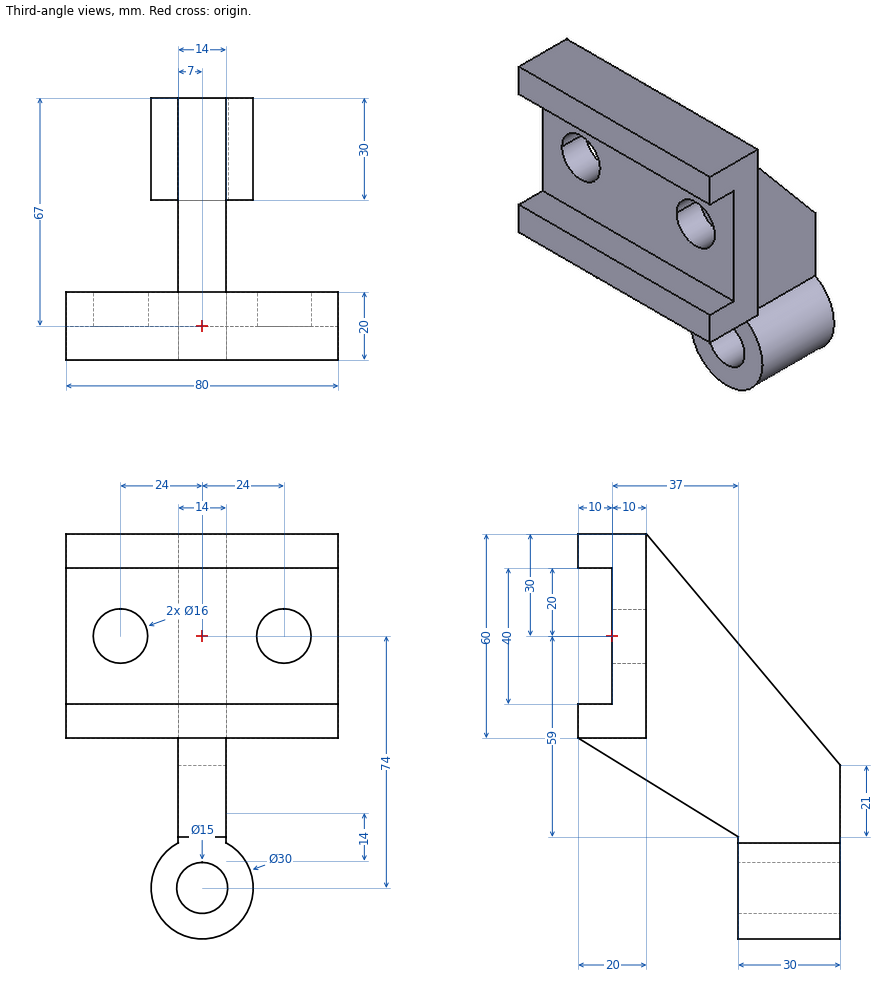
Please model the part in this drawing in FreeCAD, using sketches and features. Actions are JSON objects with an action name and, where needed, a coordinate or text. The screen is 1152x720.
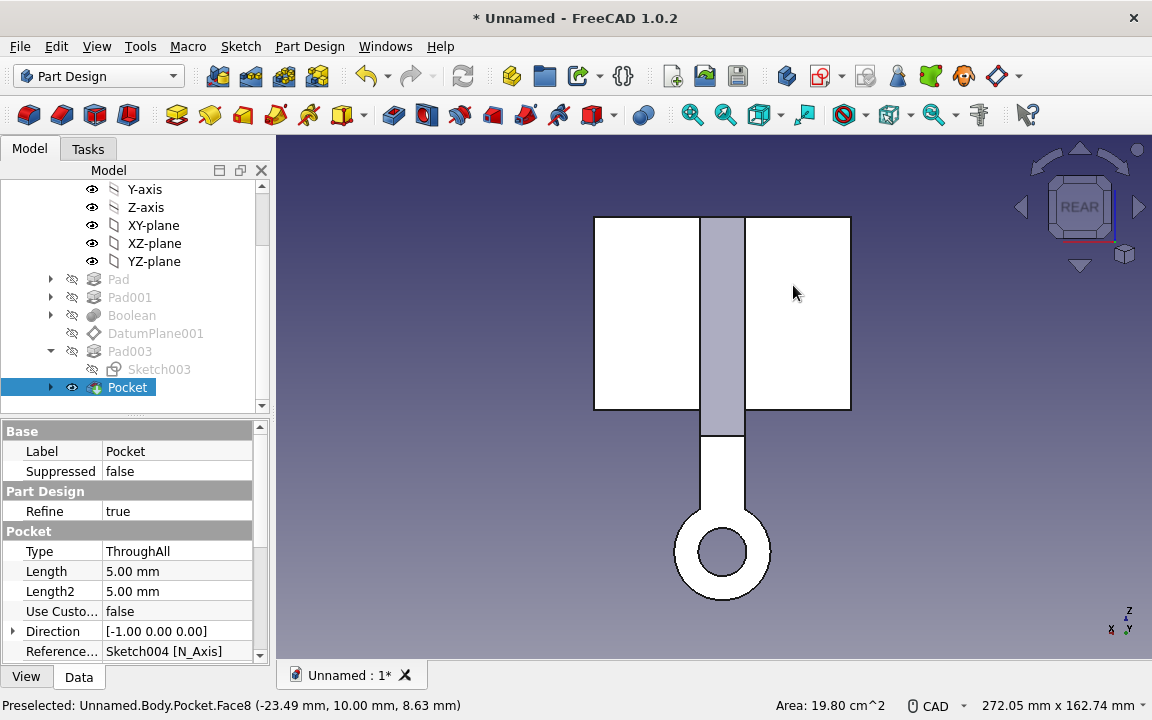
{"action": "left_click", "coordinate": [820, 76]}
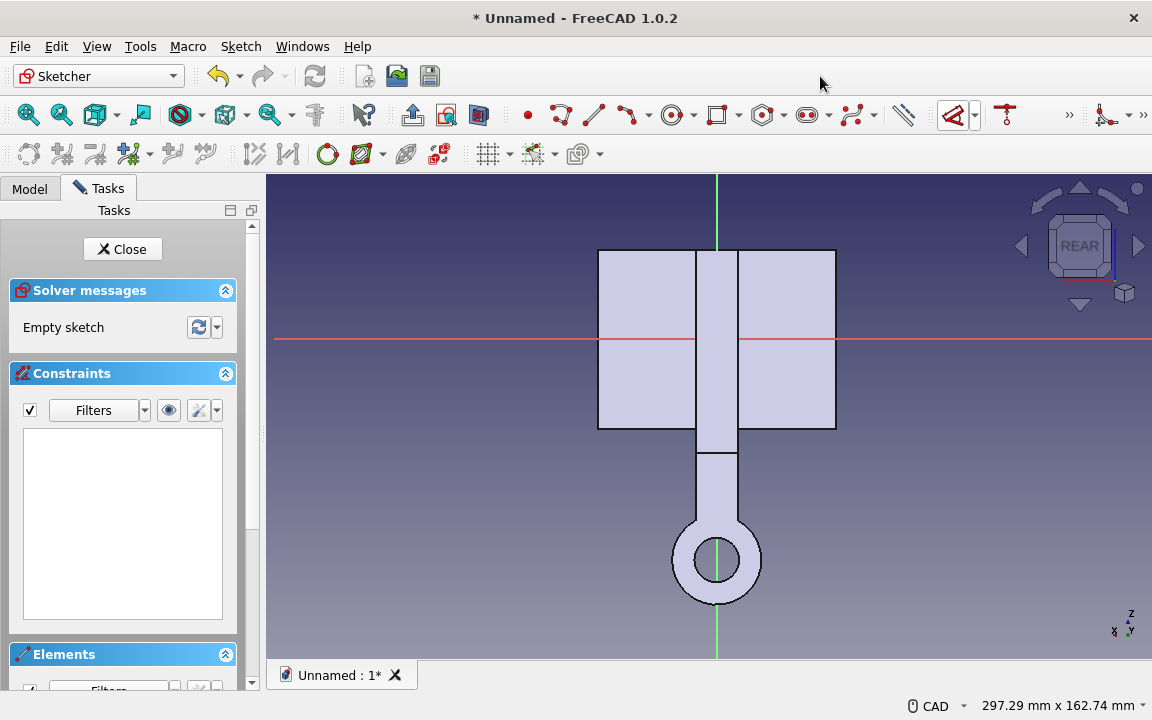
{"action": "scroll", "coordinate": [761, 295], "scroll_direction": "up", "scroll_amount": 5}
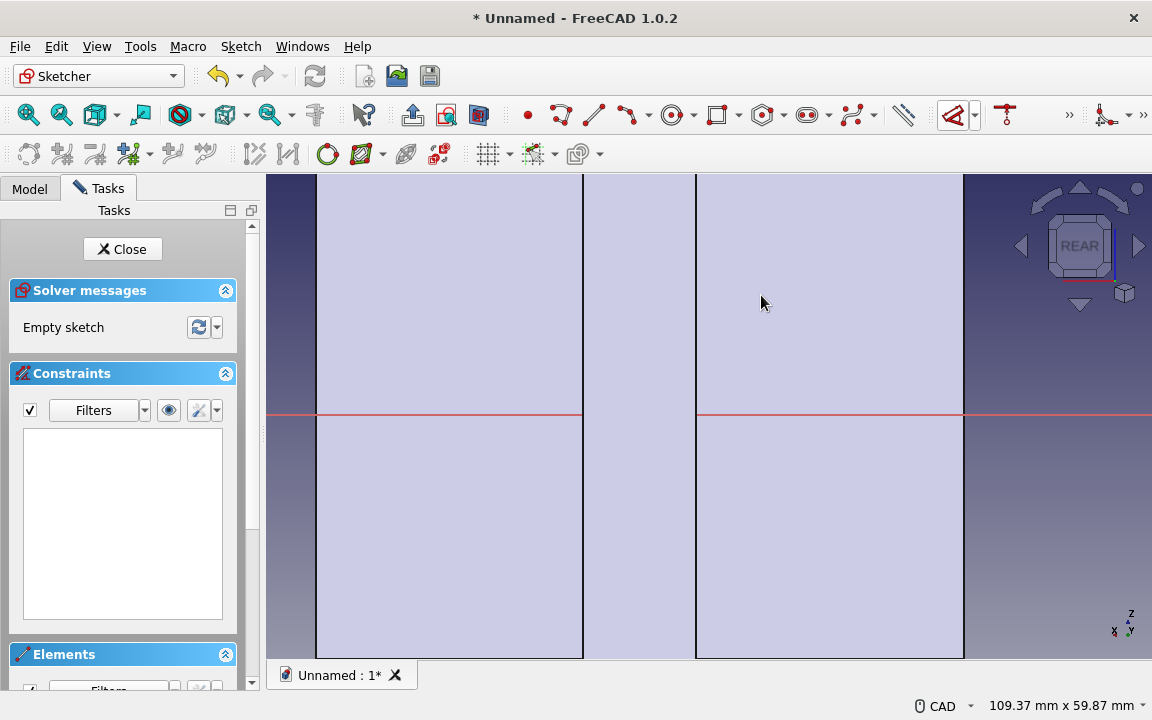
{"action": "left_click", "coordinate": [672, 116]}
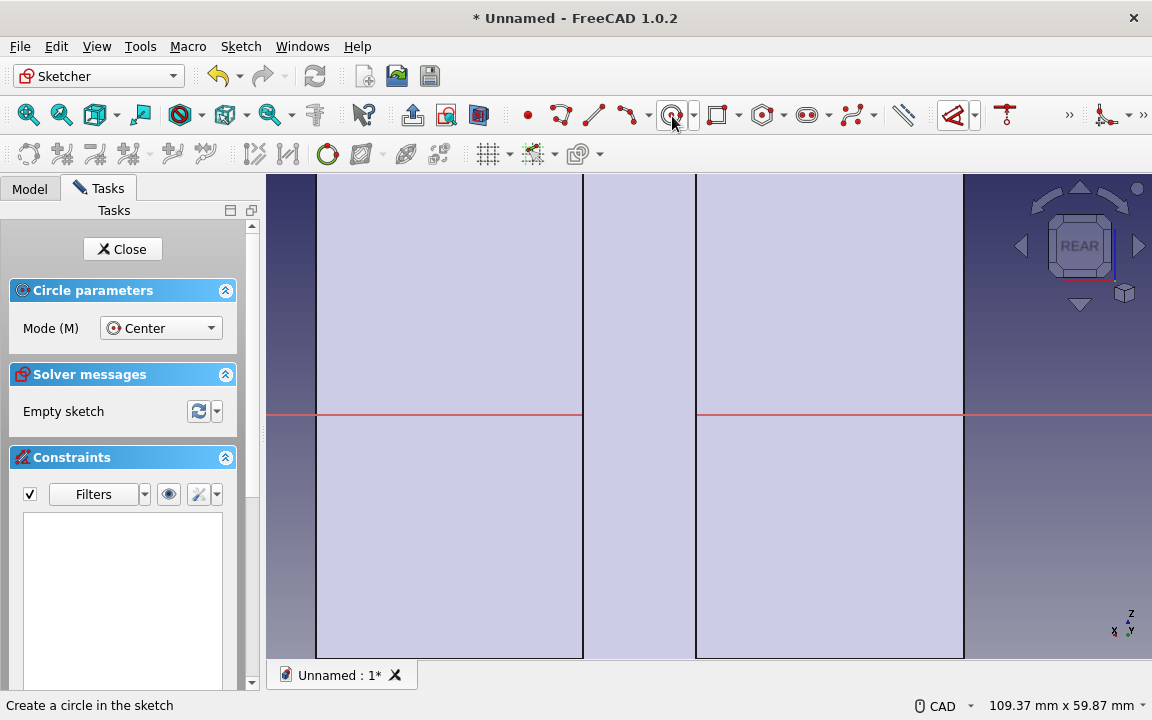
{"action": "left_click", "coordinate": [834, 415]}
{"action": "mouse_move", "coordinate": [880, 370]}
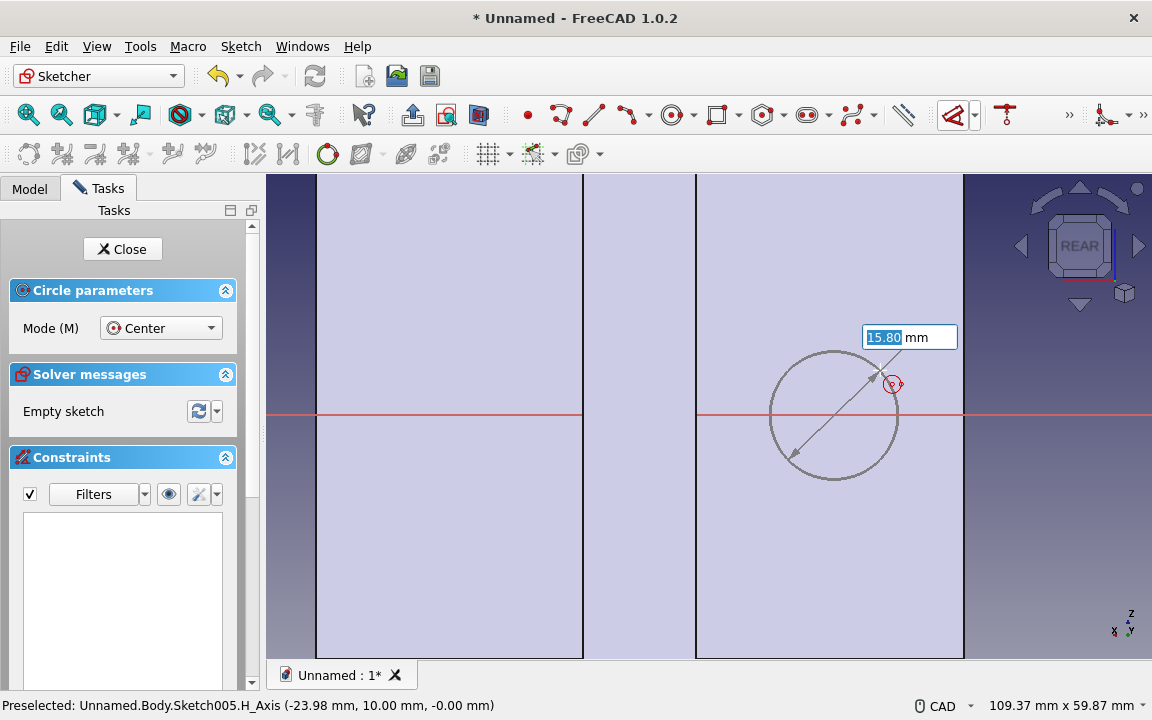
{"action": "type", "text": "16"}
{"action": "key", "text": "Return"}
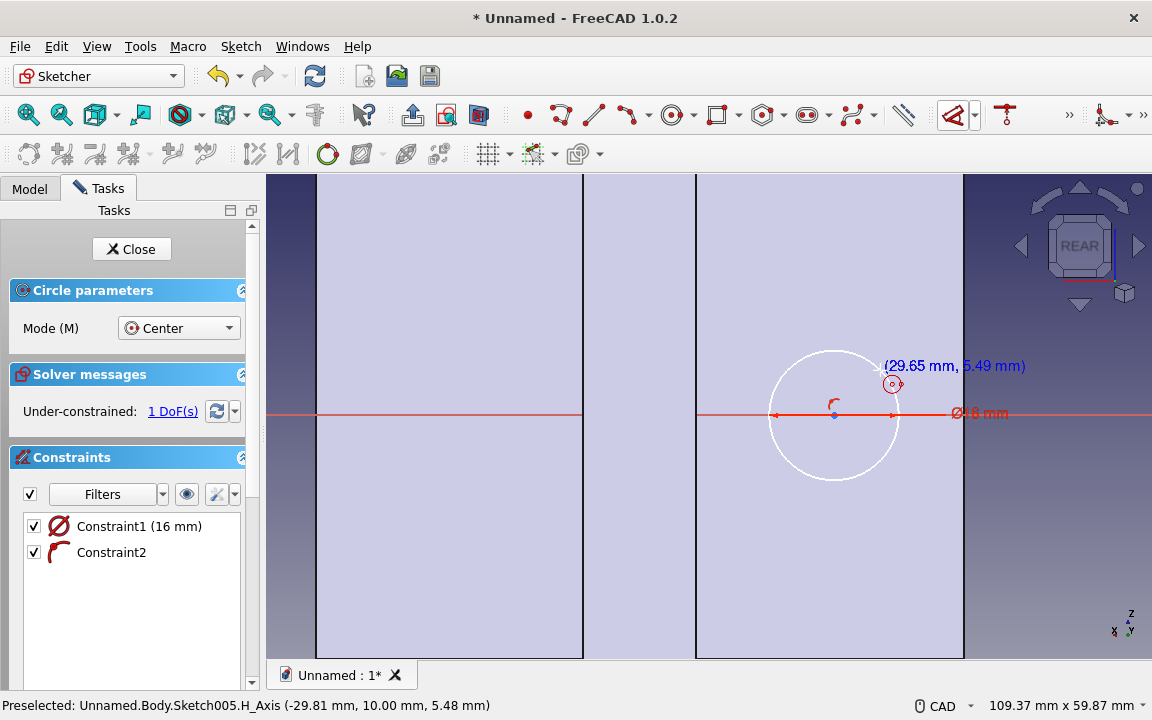
{"action": "left_click", "coordinate": [445, 415]}
{"action": "mouse_move", "coordinate": [491, 370]}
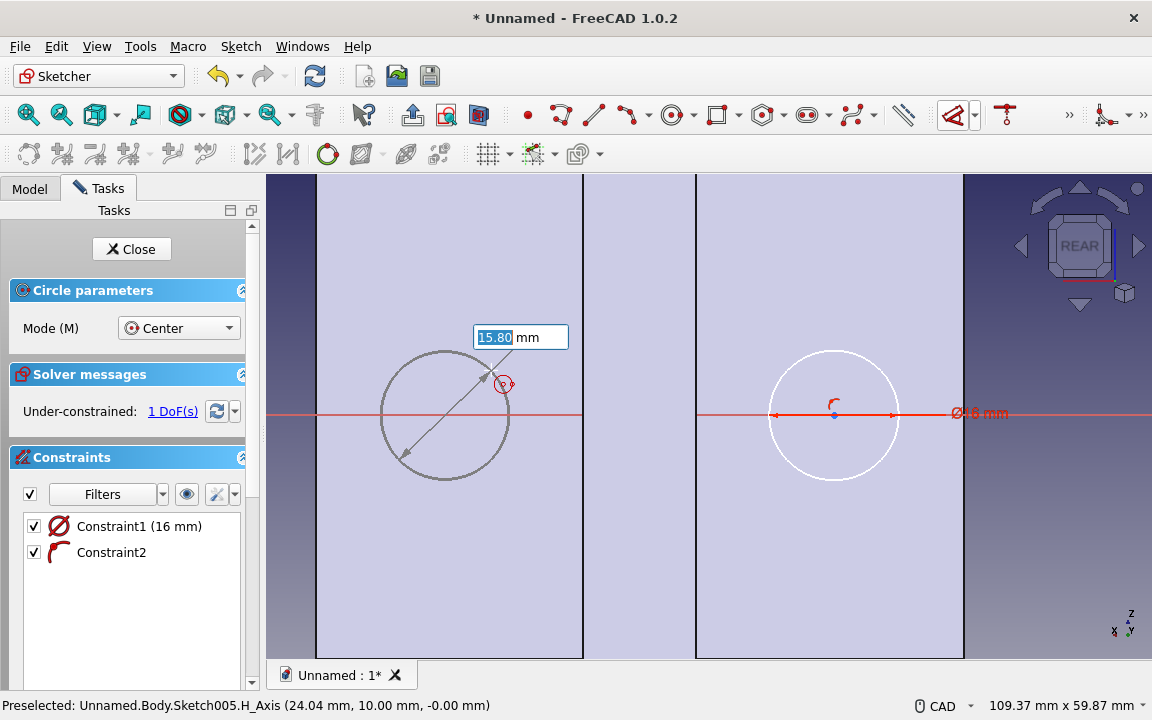
{"action": "type", "text": "16"}
{"action": "key", "text": "Return"}
{"action": "key", "text": "Escape"}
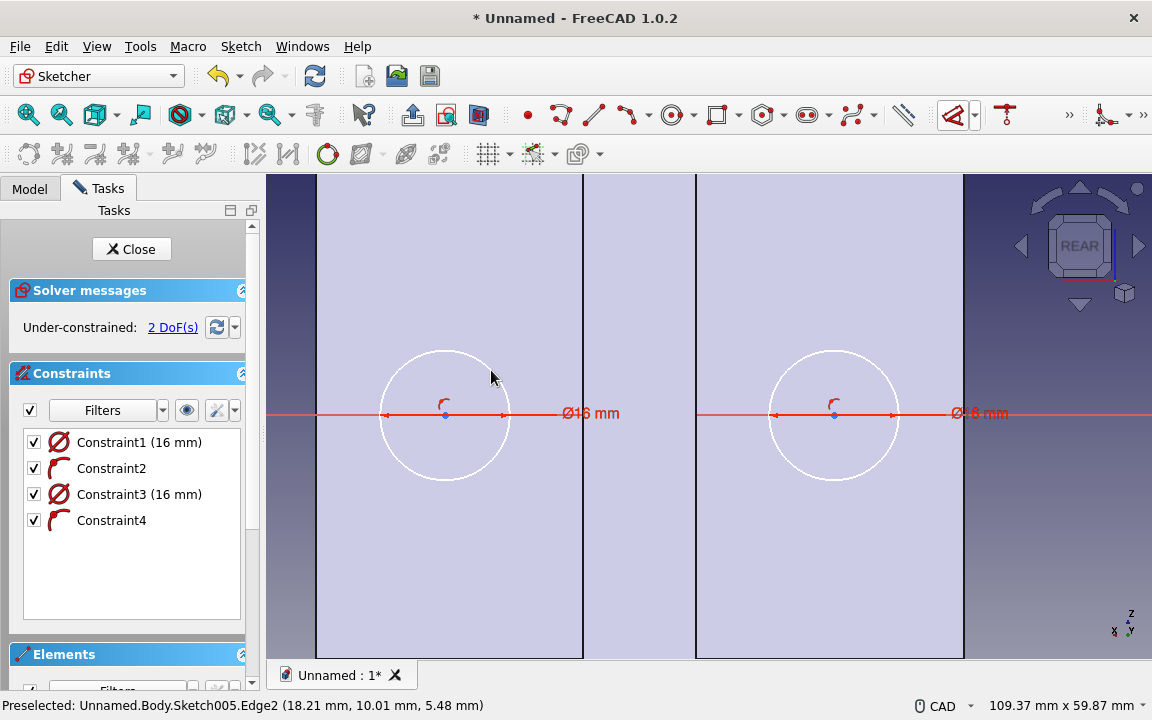
{"action": "left_click", "coordinate": [834, 415]}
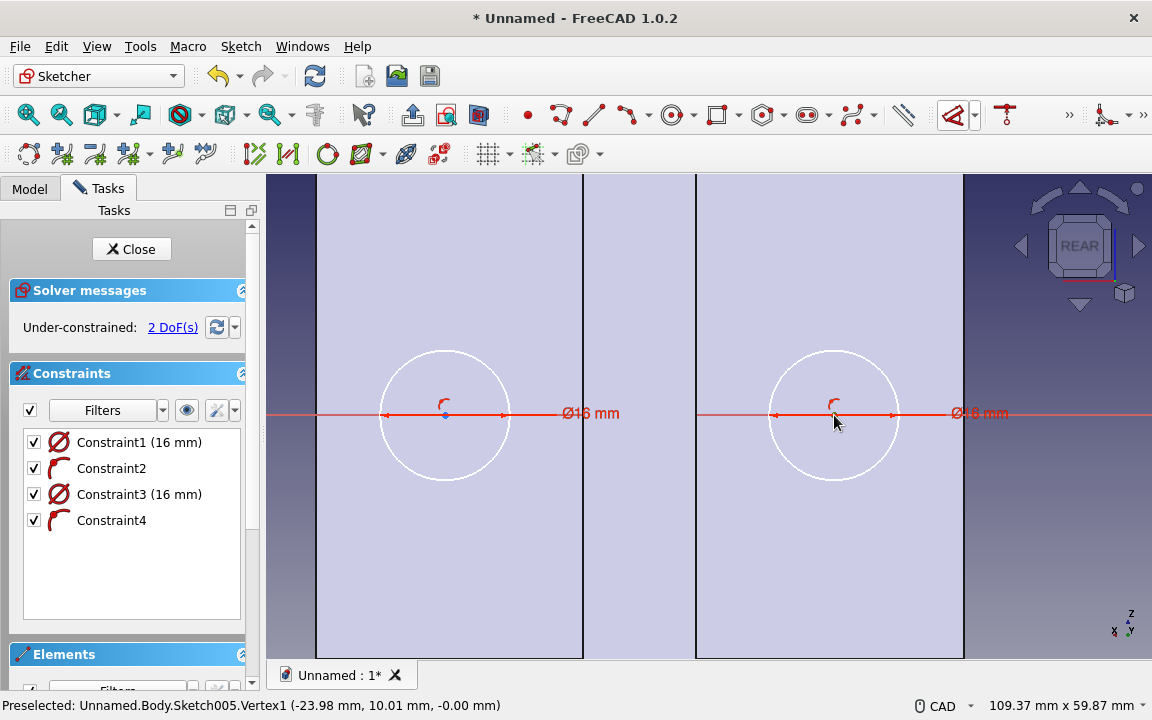
{"action": "left_click", "coordinate": [974, 116]}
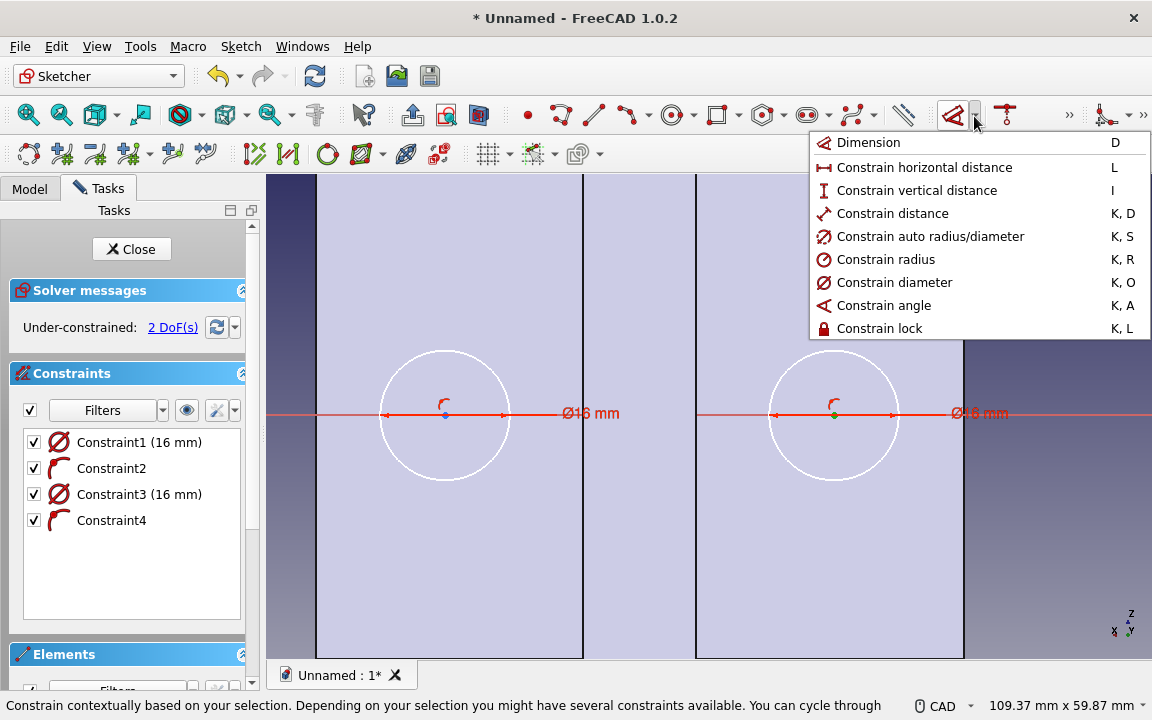
{"action": "left_click", "coordinate": [980, 168]}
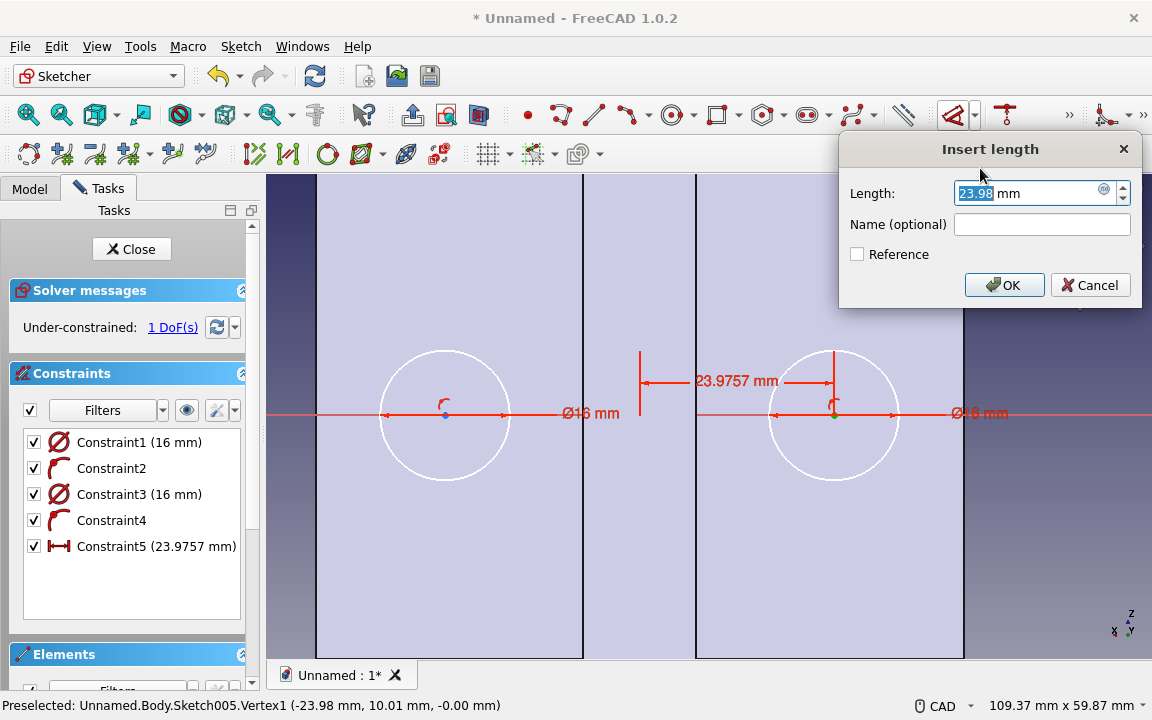
{"action": "type", "text": "24"}
{"action": "key", "text": "Return"}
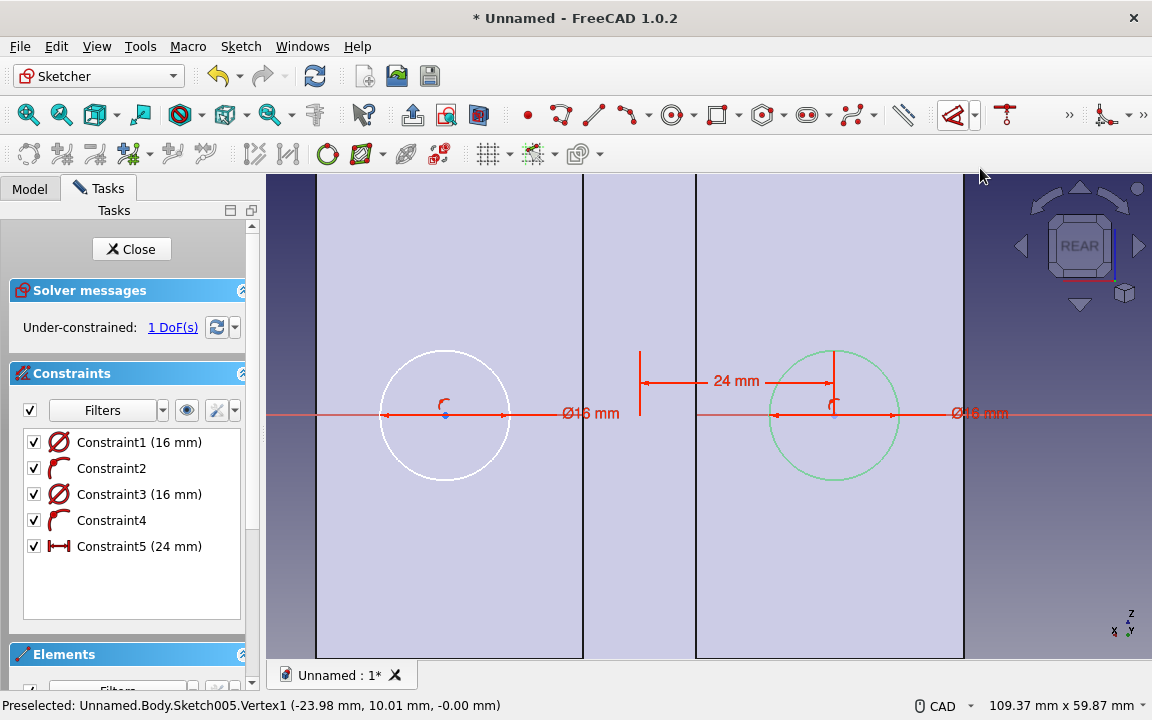
{"action": "left_click", "coordinate": [445, 415]}